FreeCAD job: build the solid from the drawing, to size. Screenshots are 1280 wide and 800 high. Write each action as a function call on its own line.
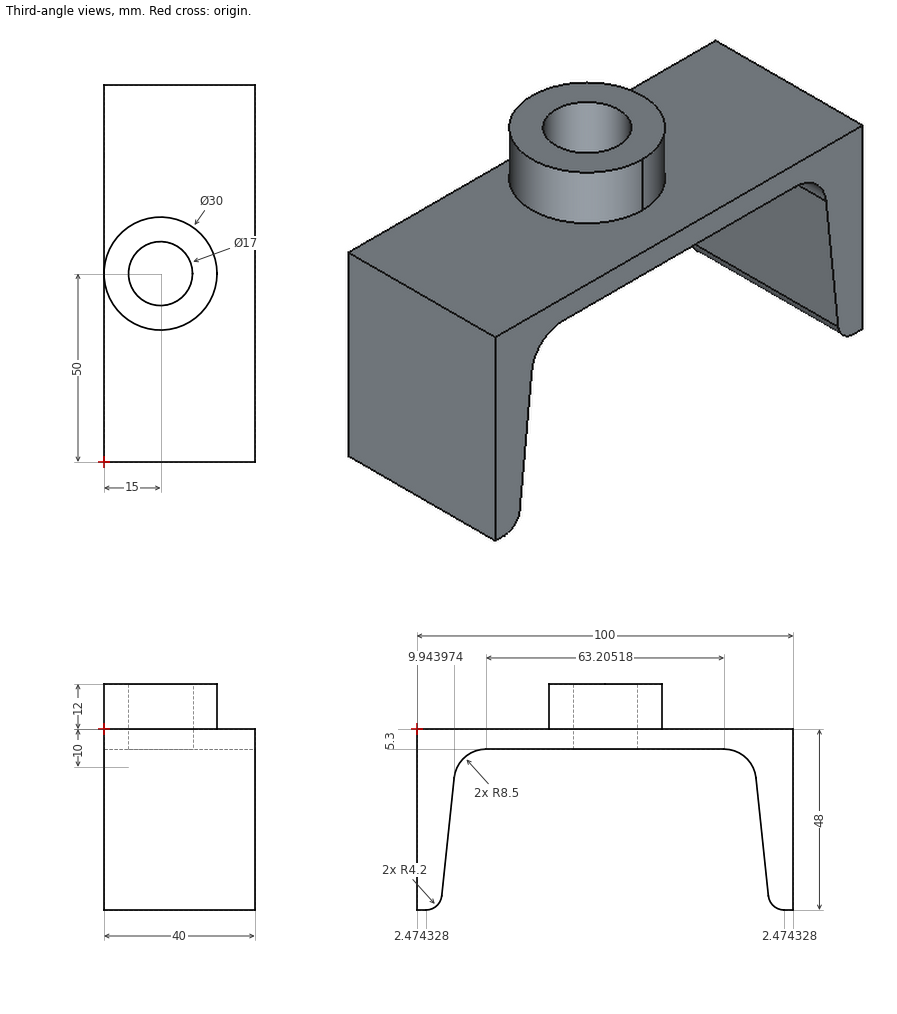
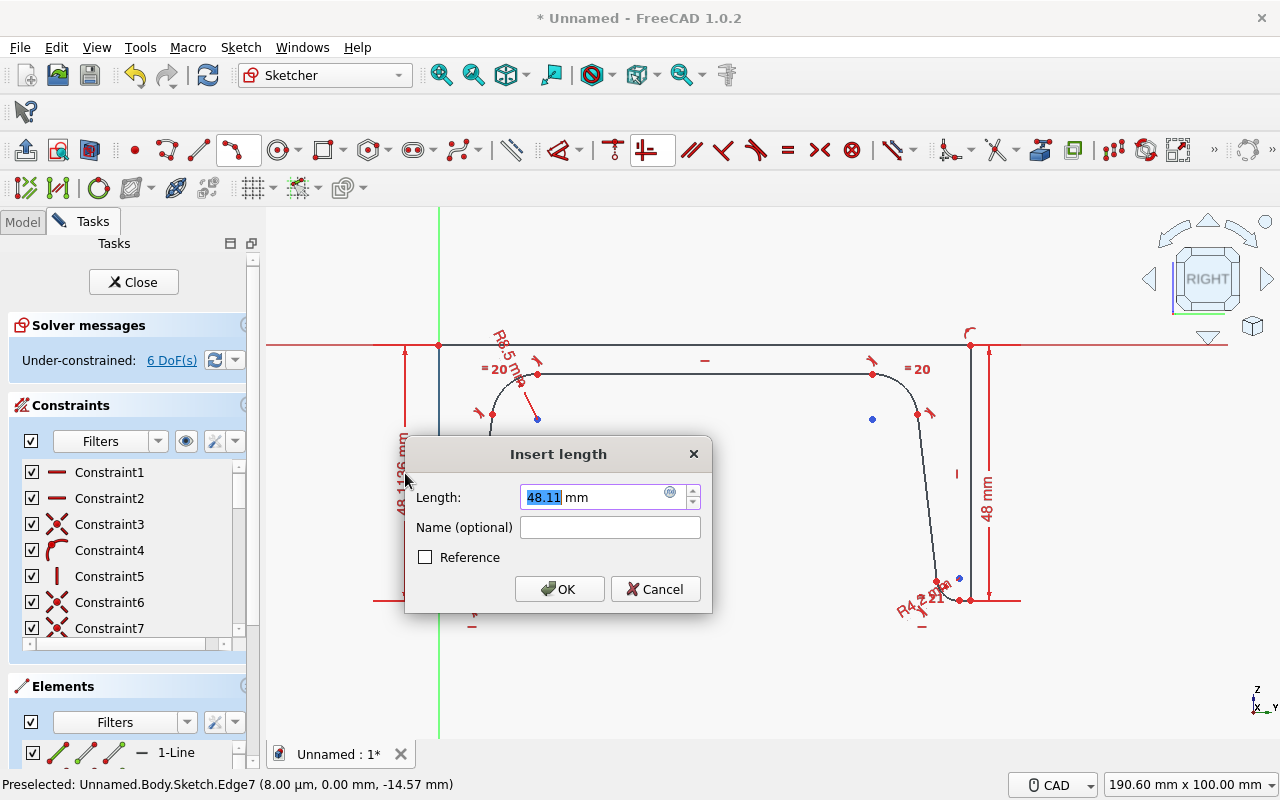
text(48)
key(Return)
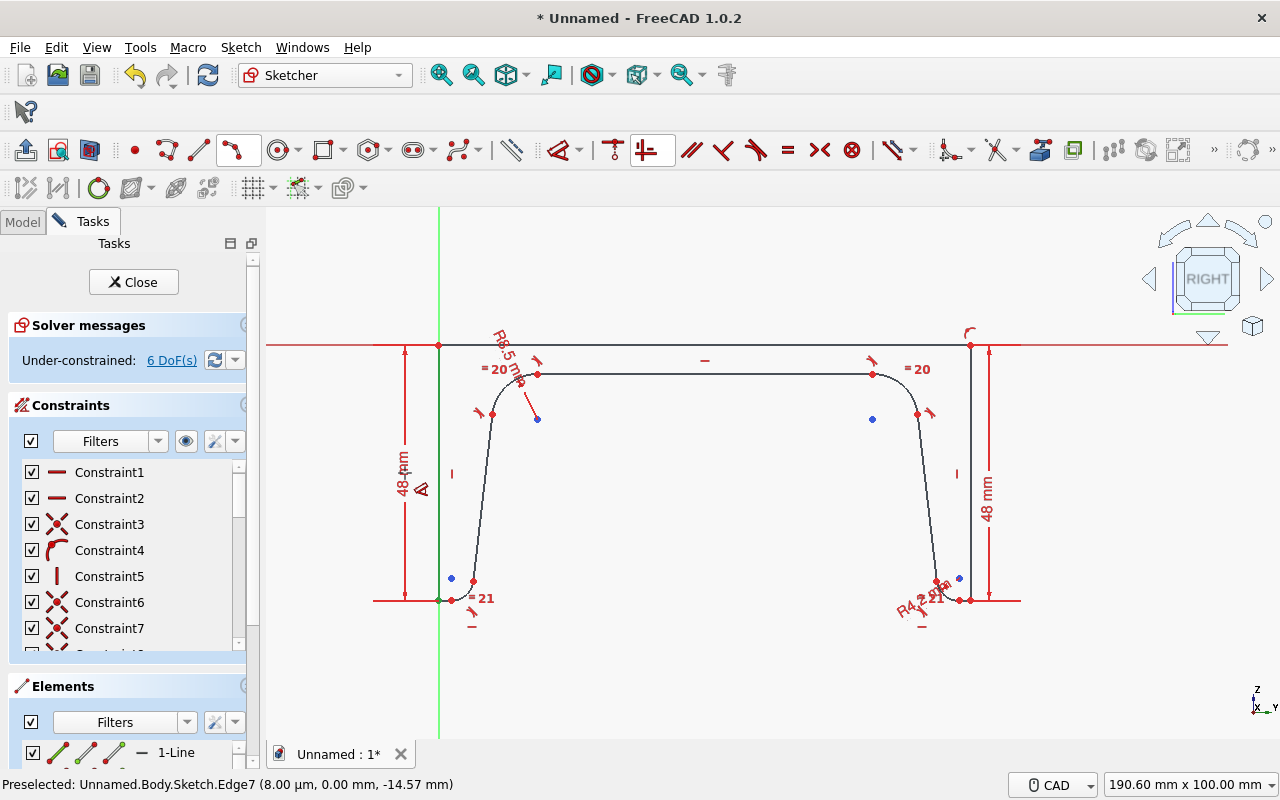
click(811, 345)
click(705, 311)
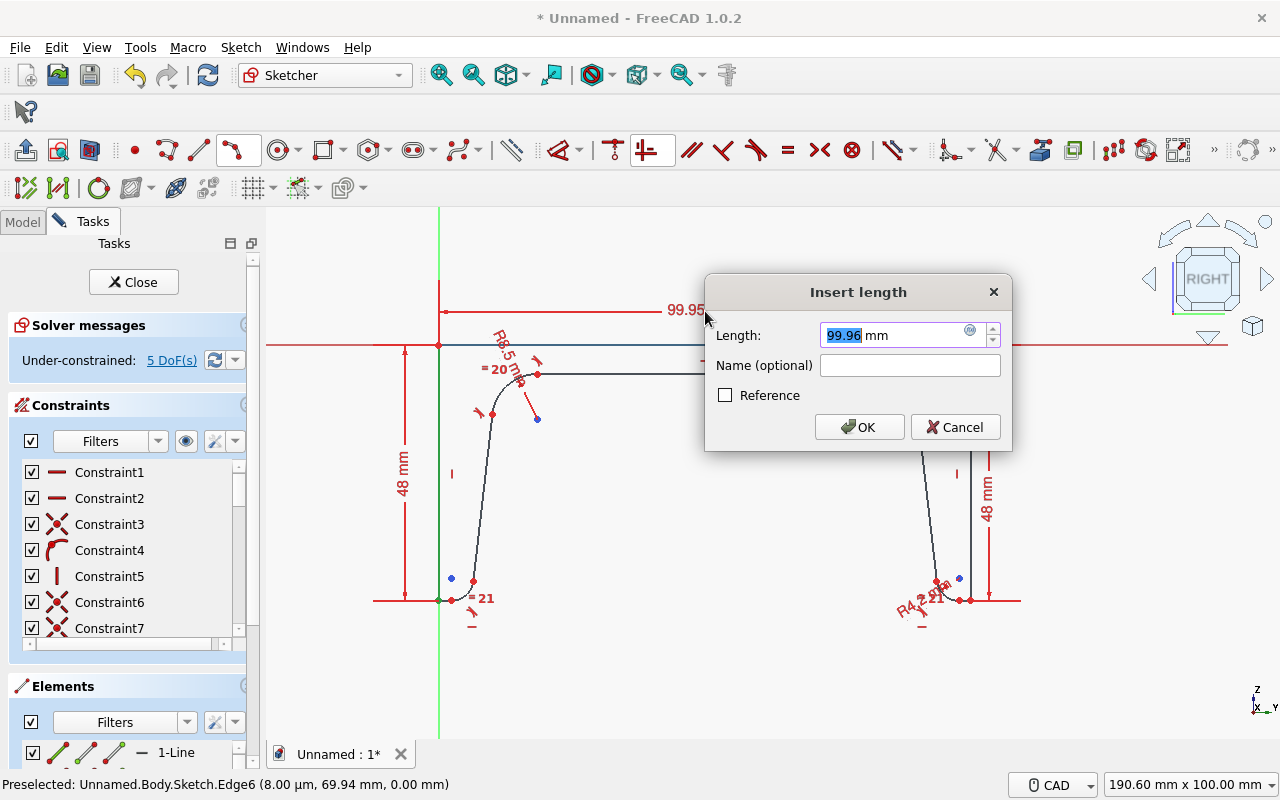
text(100)
key(Return)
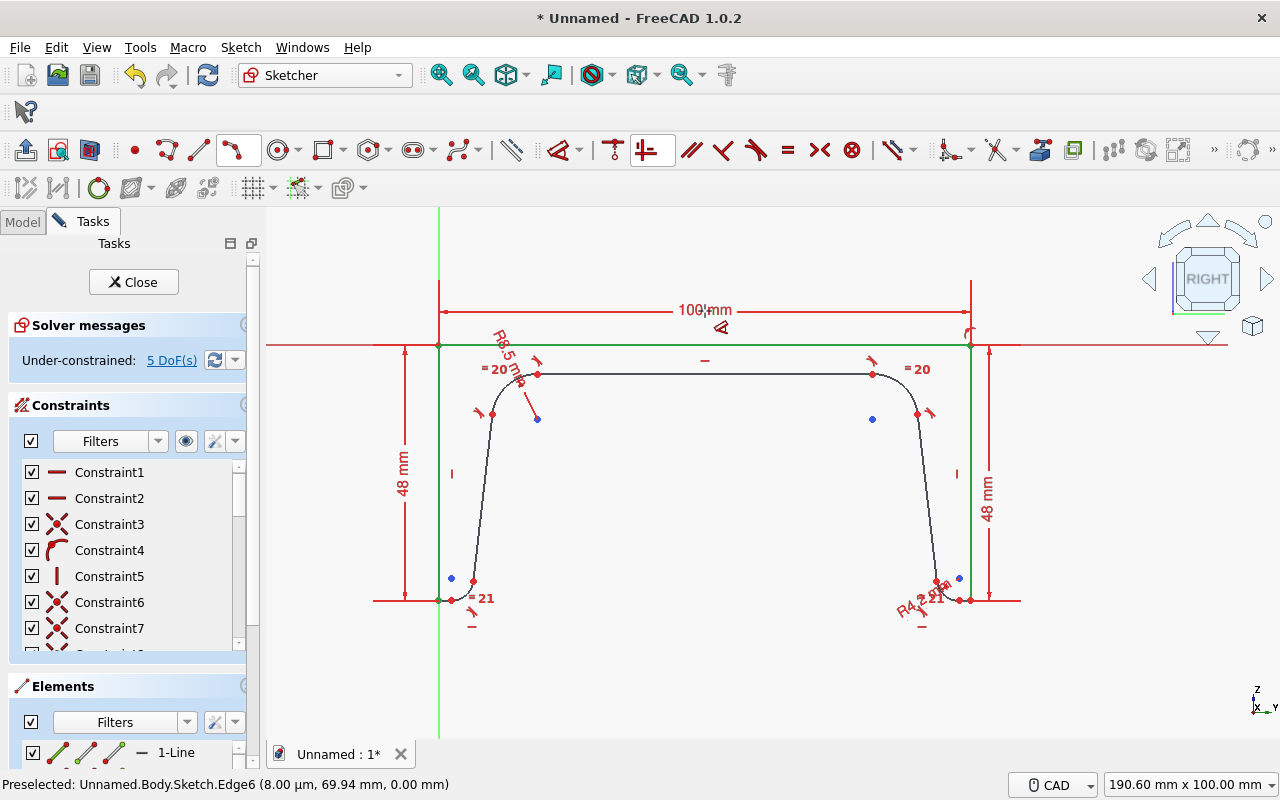
scroll(537, 374, up, 2)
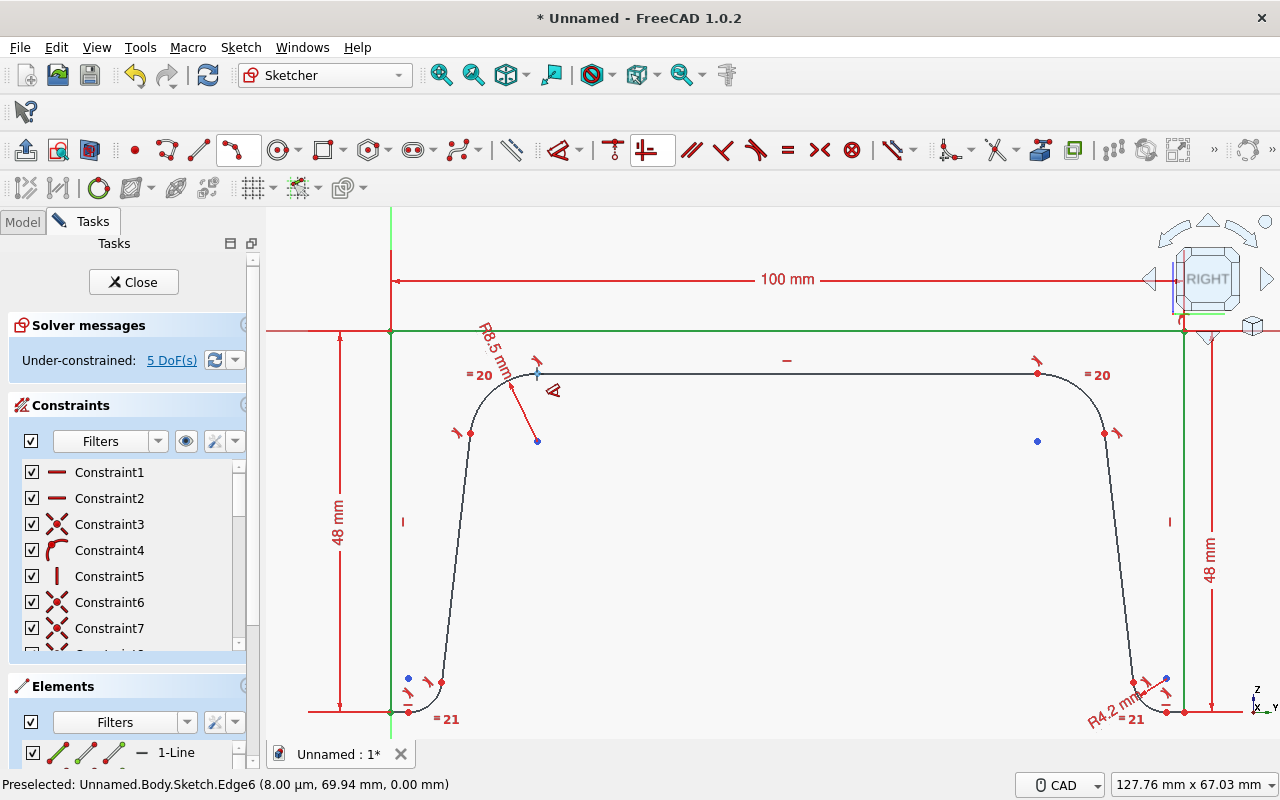
click(537, 374)
click(357, 353)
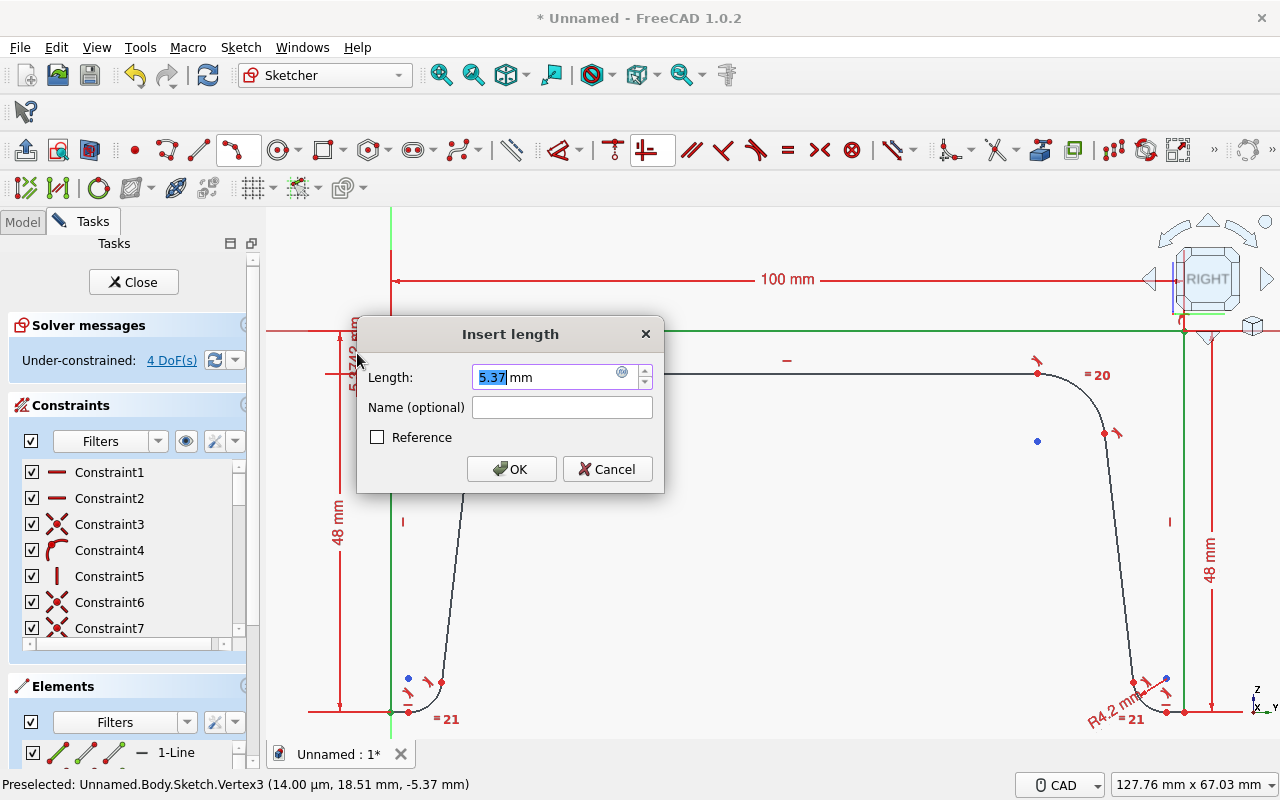
text(5.3)
key(Return)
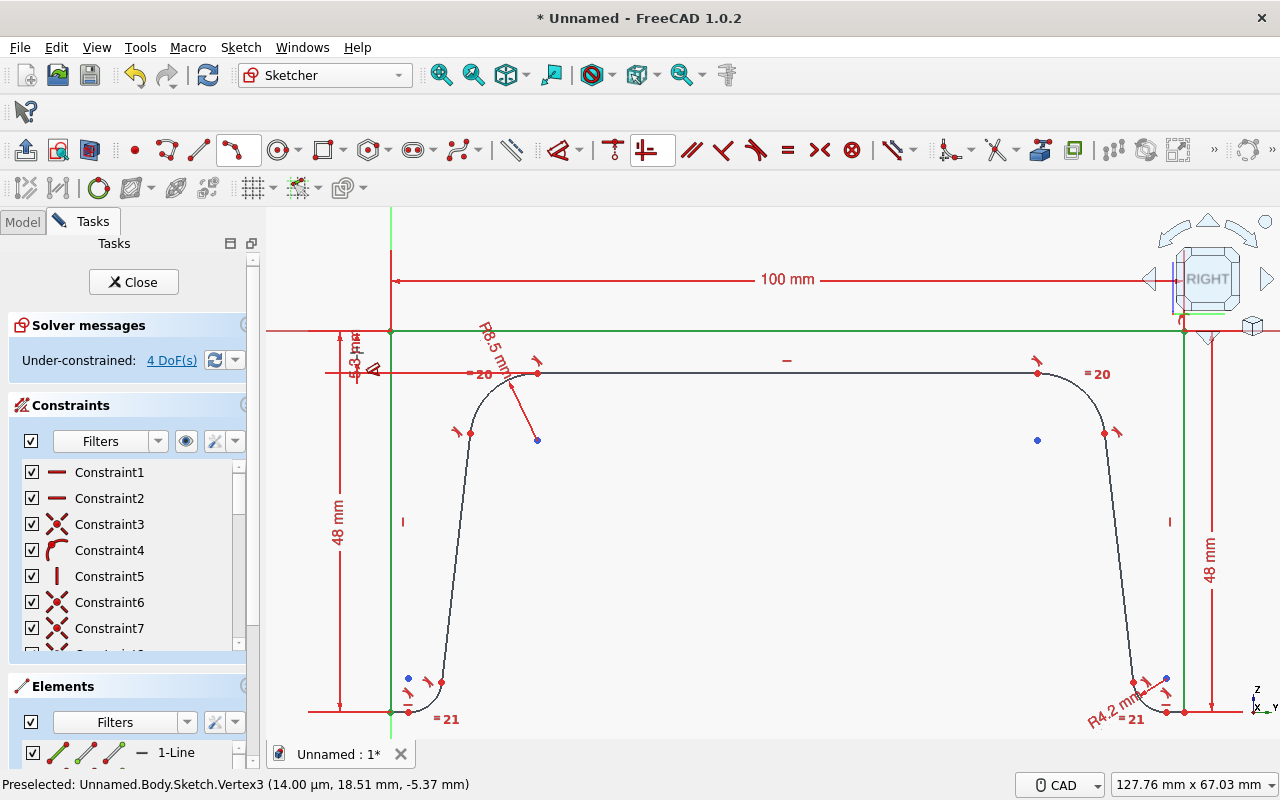
click(688, 373)
click(788, 407)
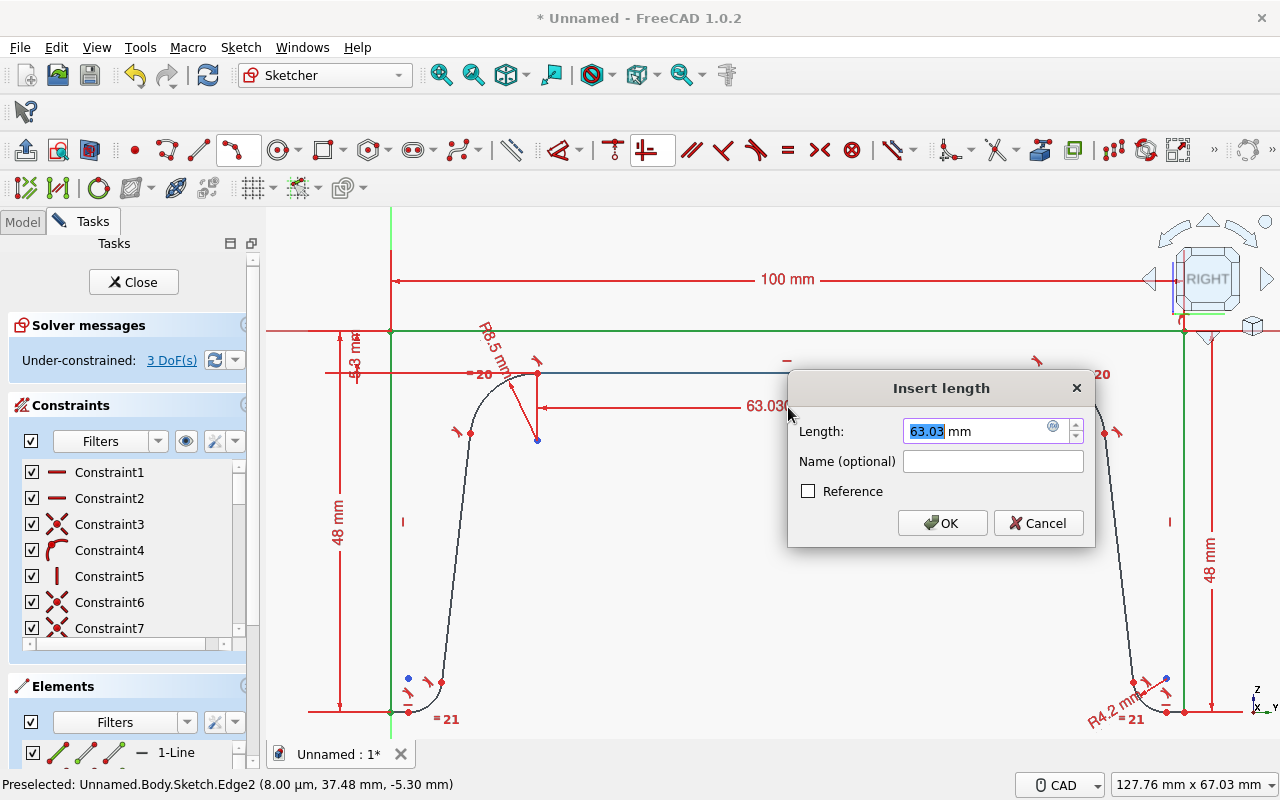
text(63.20518)
key(Return)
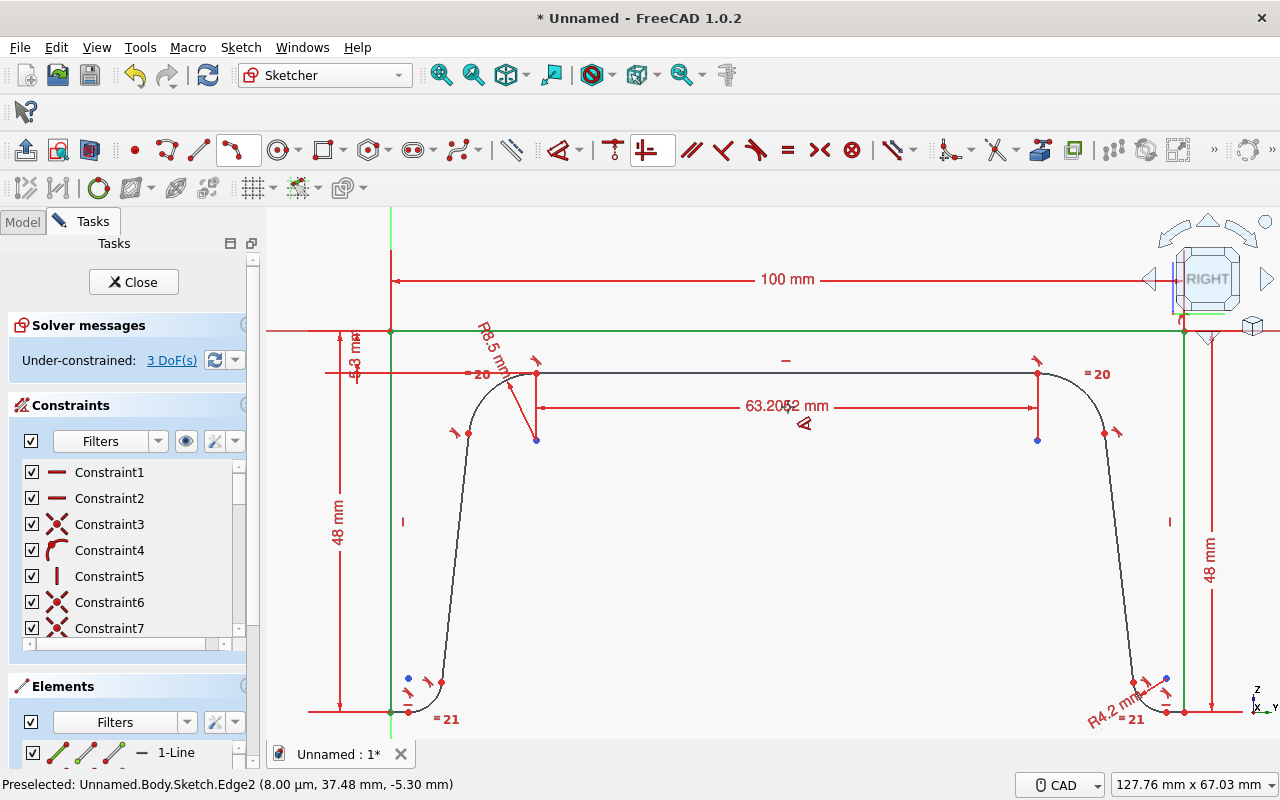
scroll(536, 374, down, 2)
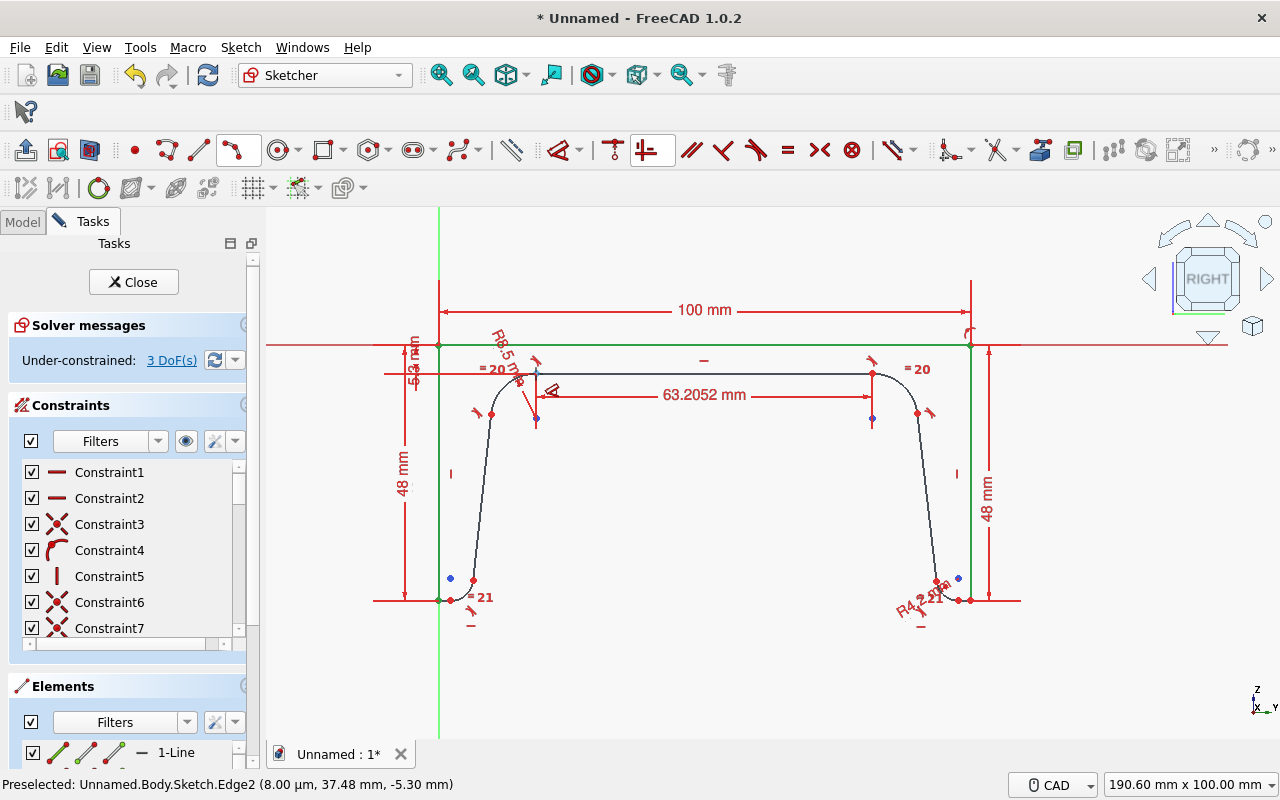
scroll(965, 601, up, 6)